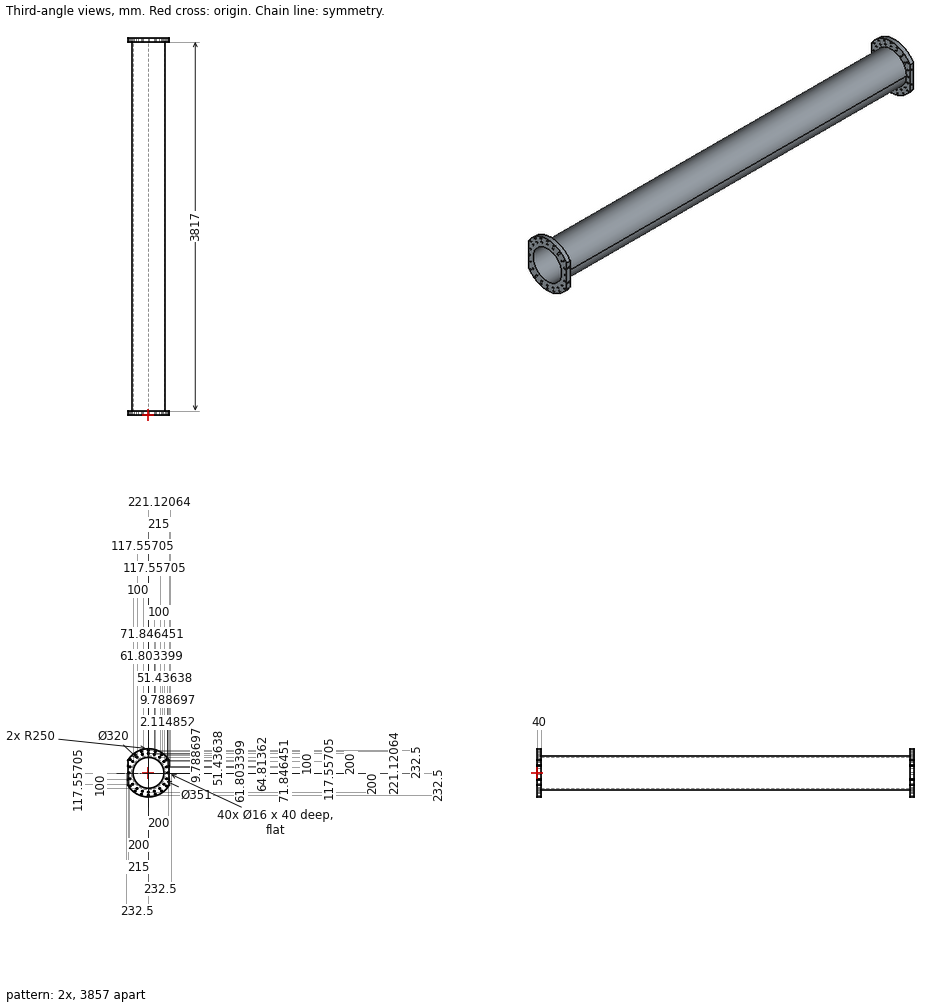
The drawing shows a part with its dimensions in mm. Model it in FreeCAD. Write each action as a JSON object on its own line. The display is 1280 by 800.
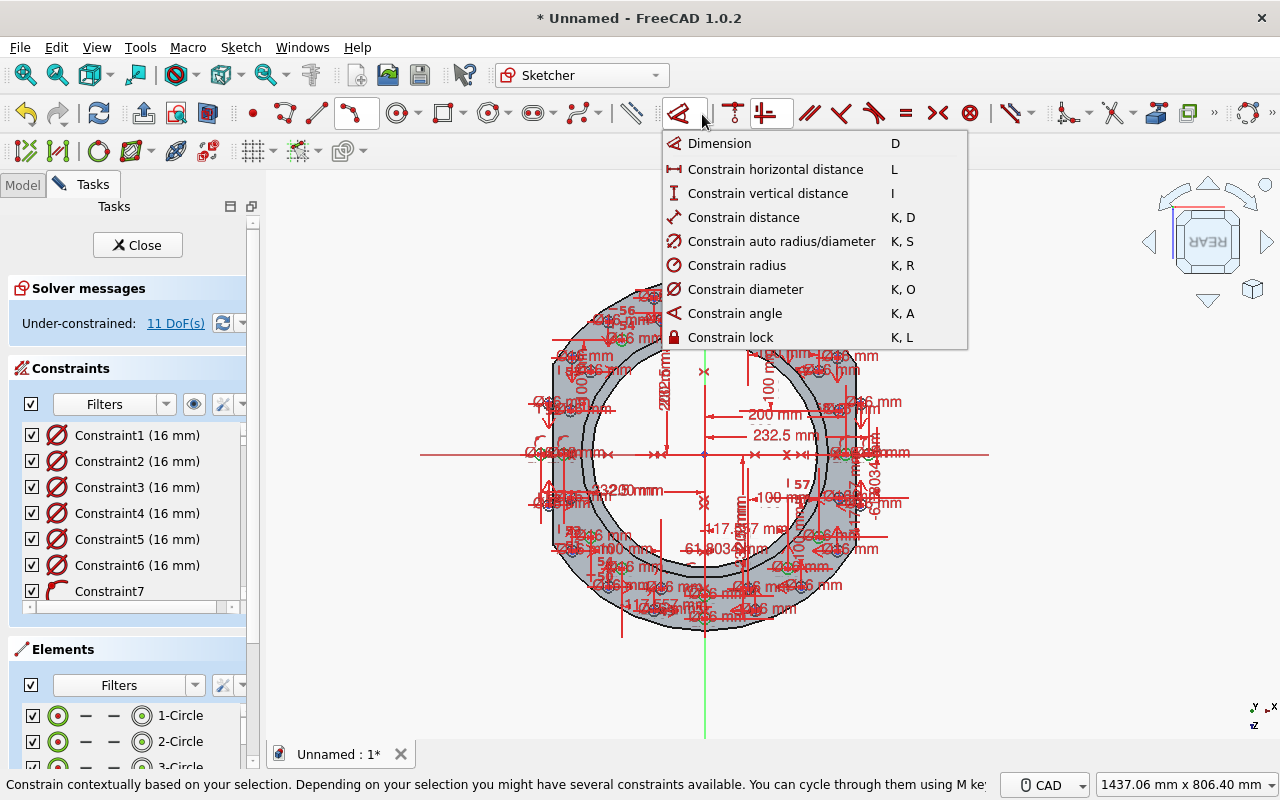
{"action": "left_click", "coordinate": [815, 193]}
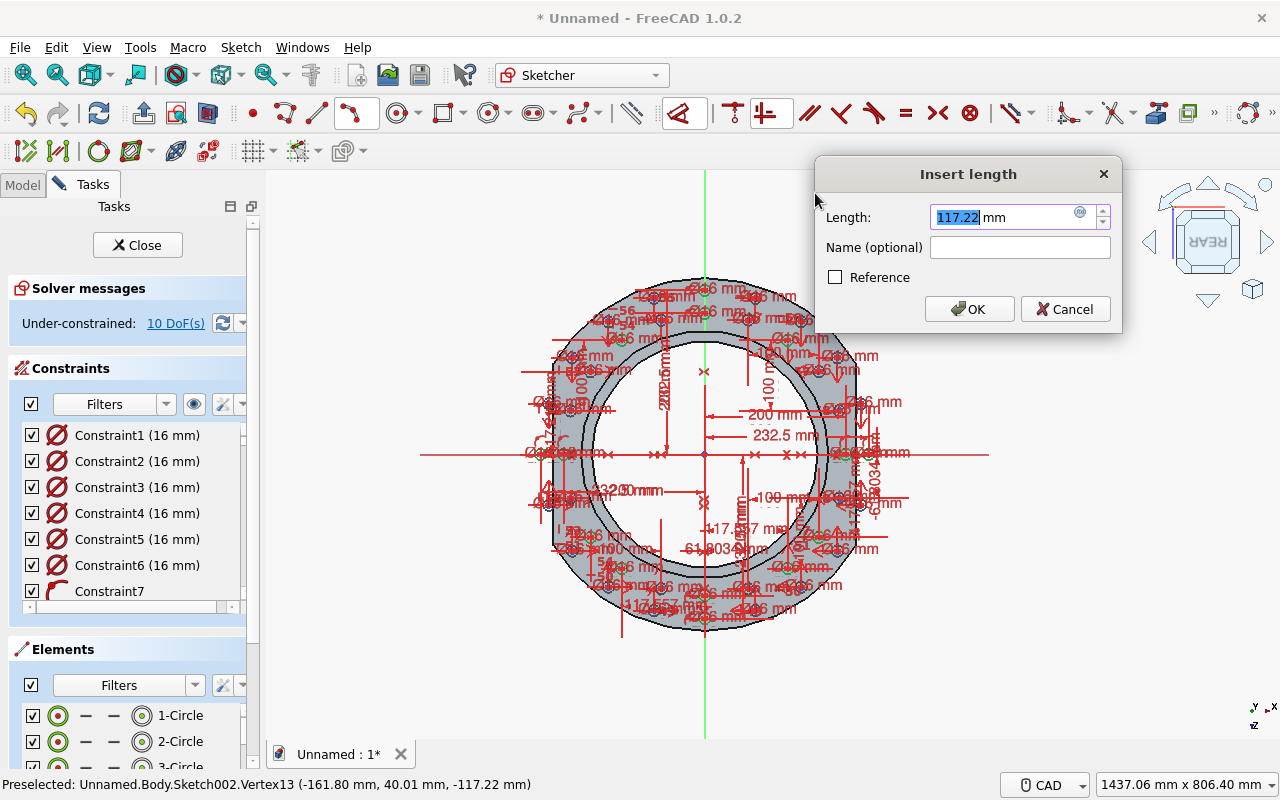
{"action": "type", "text": "117.55705"}
{"action": "key", "text": "Return"}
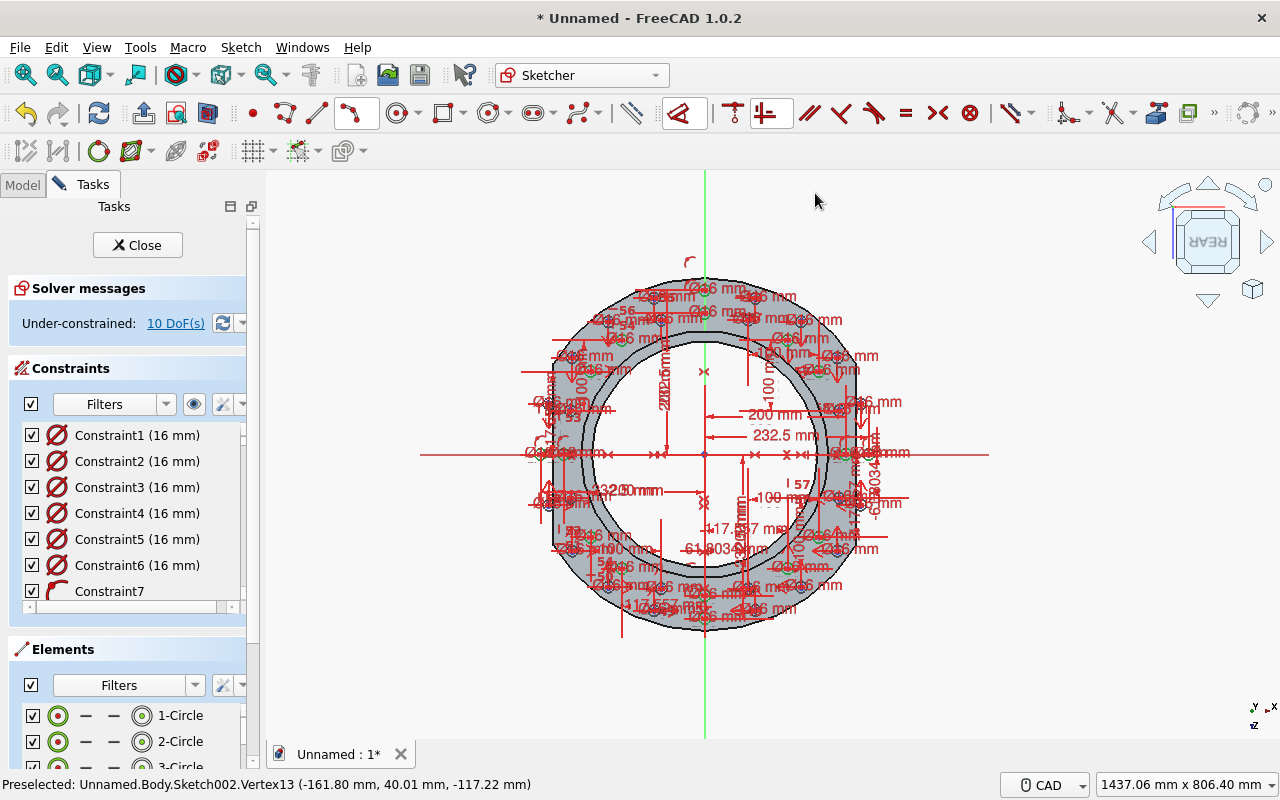
{"action": "left_click", "coordinate": [861, 505]}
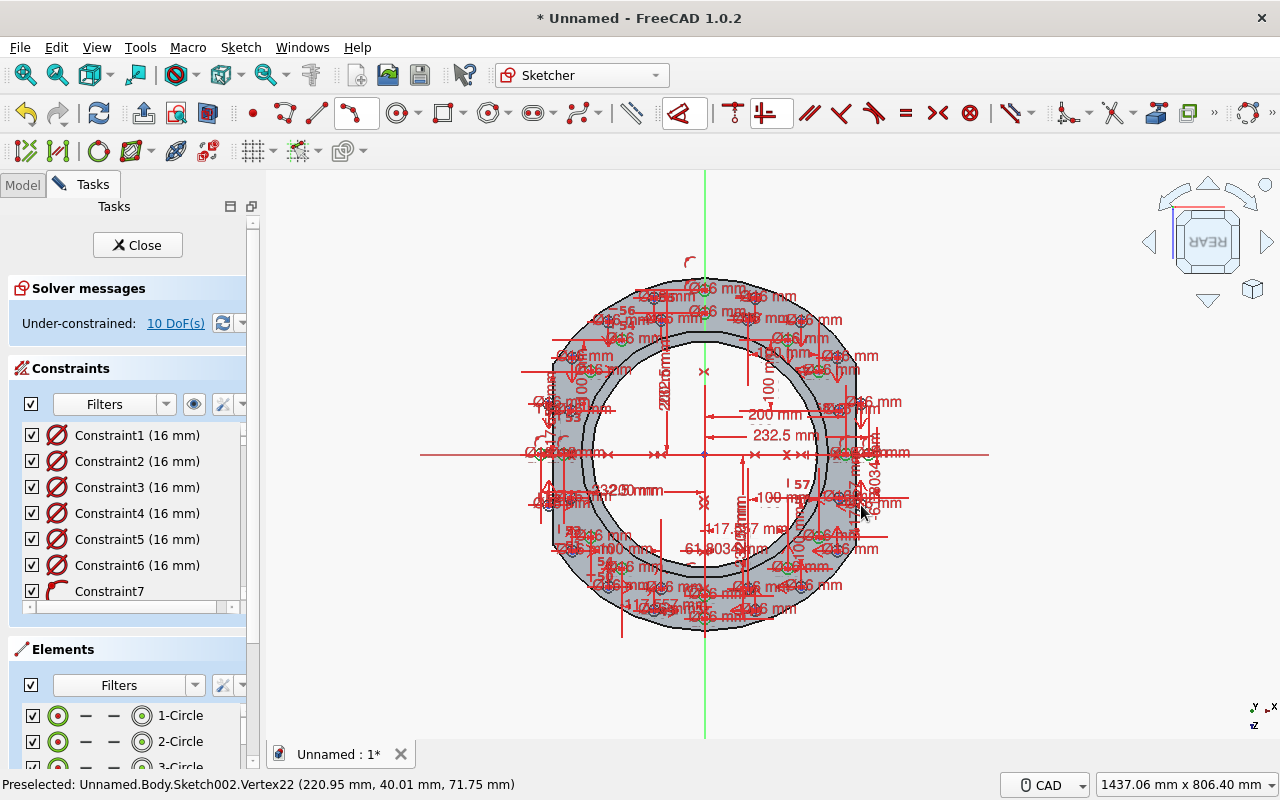
{"action": "left_click", "coordinate": [702, 114]}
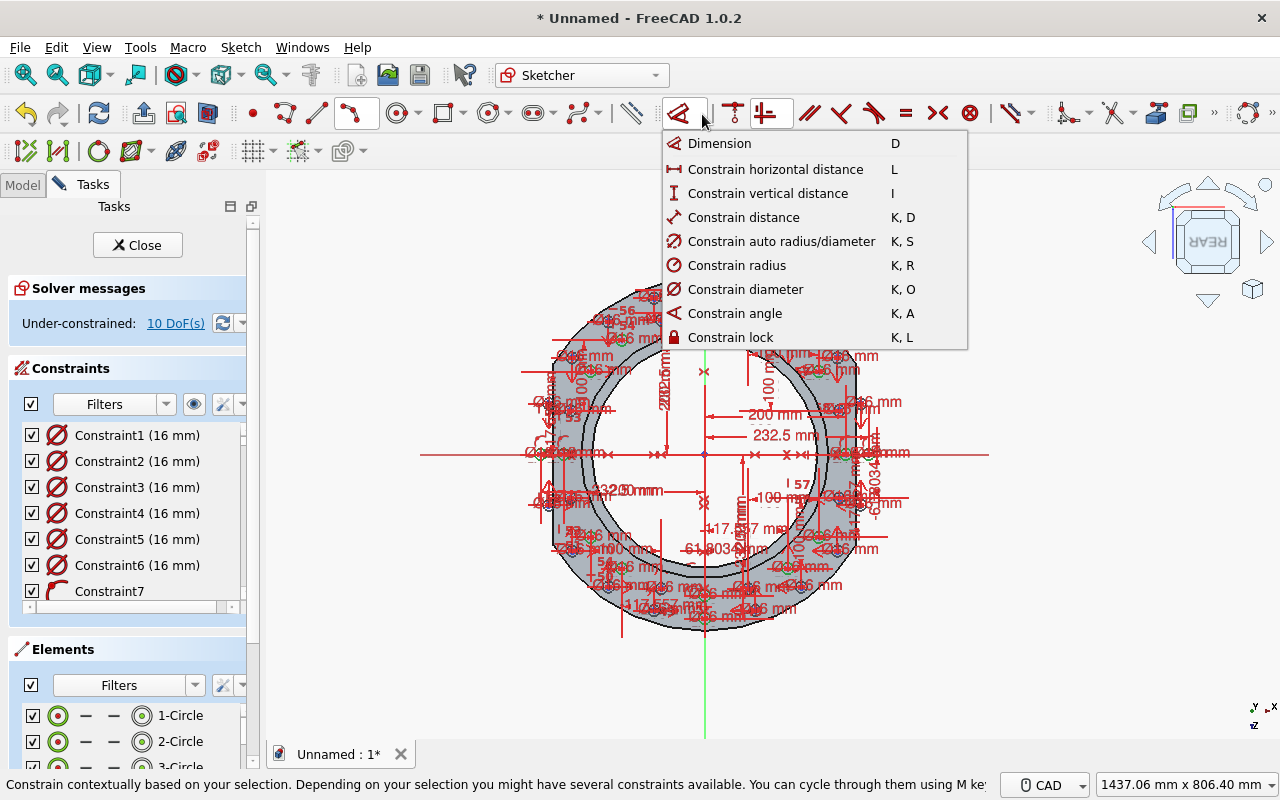
{"action": "left_click", "coordinate": [815, 169]}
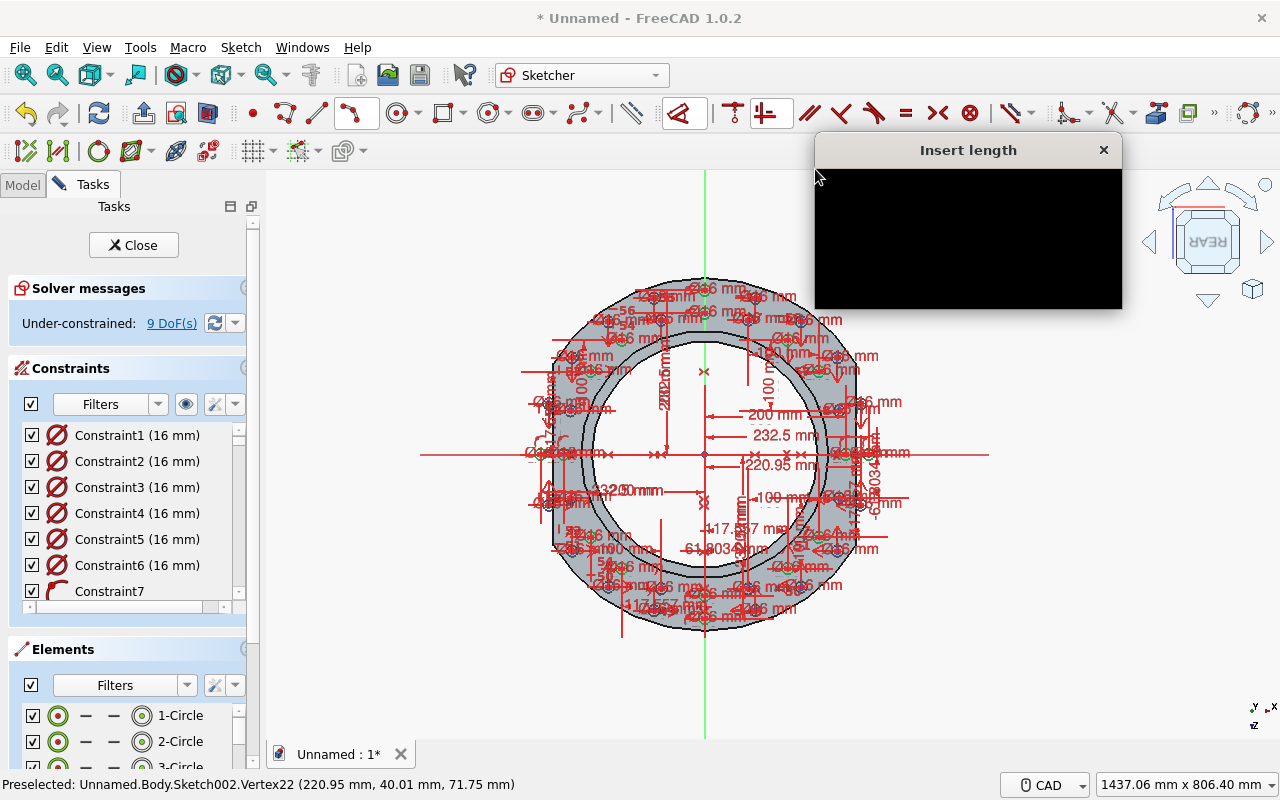
{"action": "type", "text": "221.12064"}
{"action": "key", "text": "Return"}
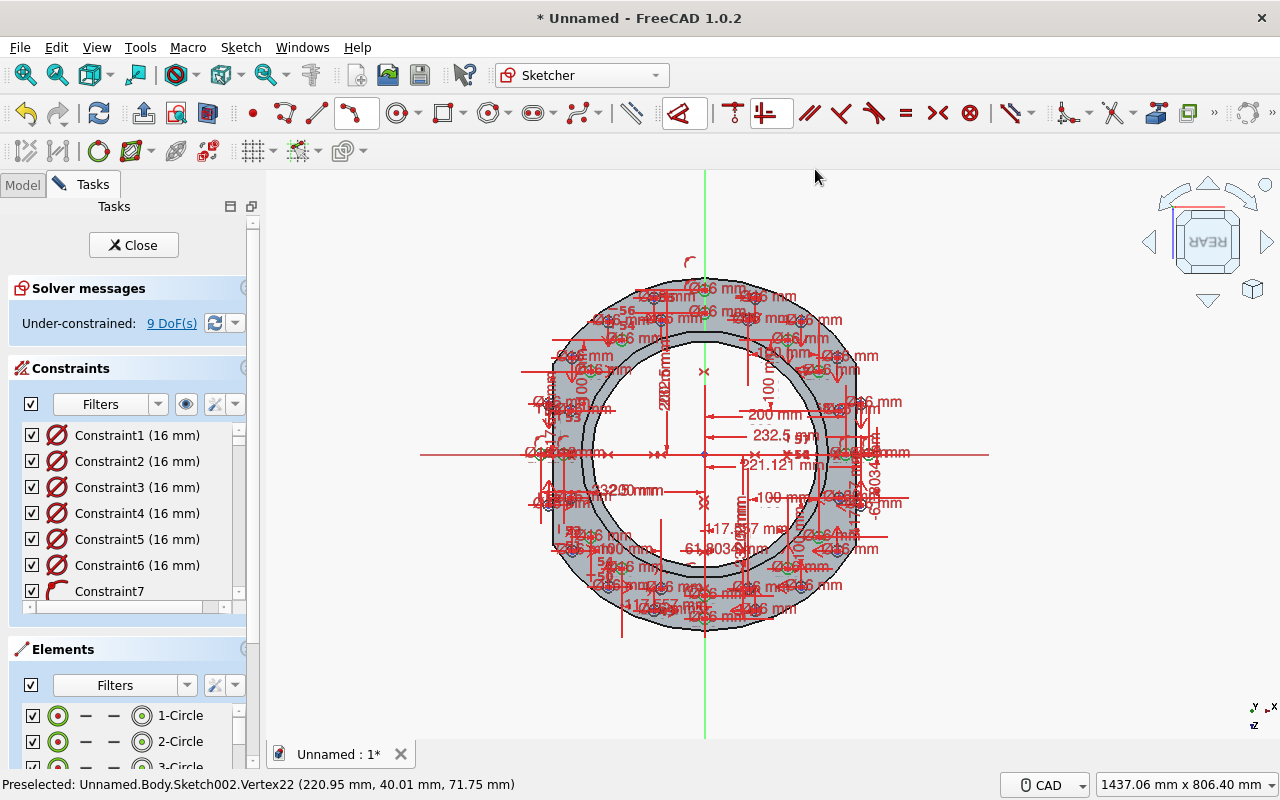
{"action": "left_click", "coordinate": [861, 505]}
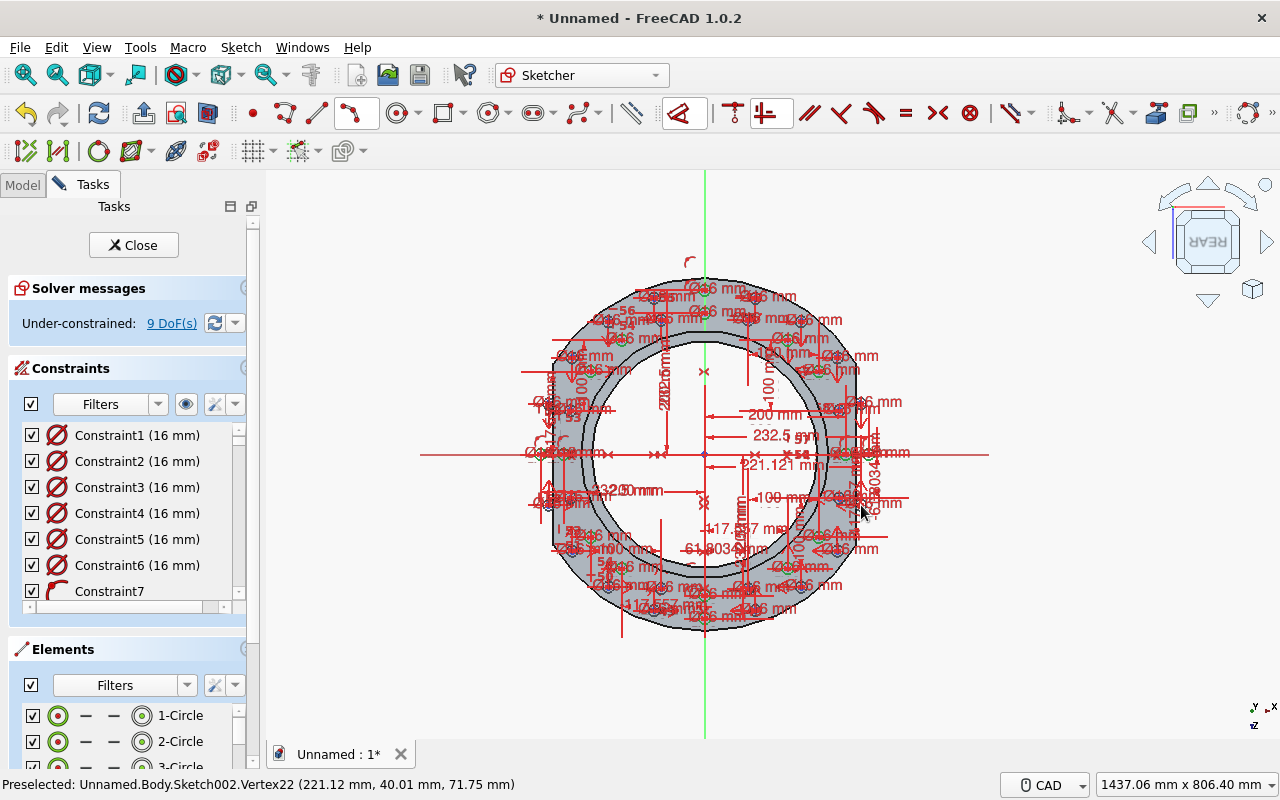
{"action": "left_click", "coordinate": [702, 114]}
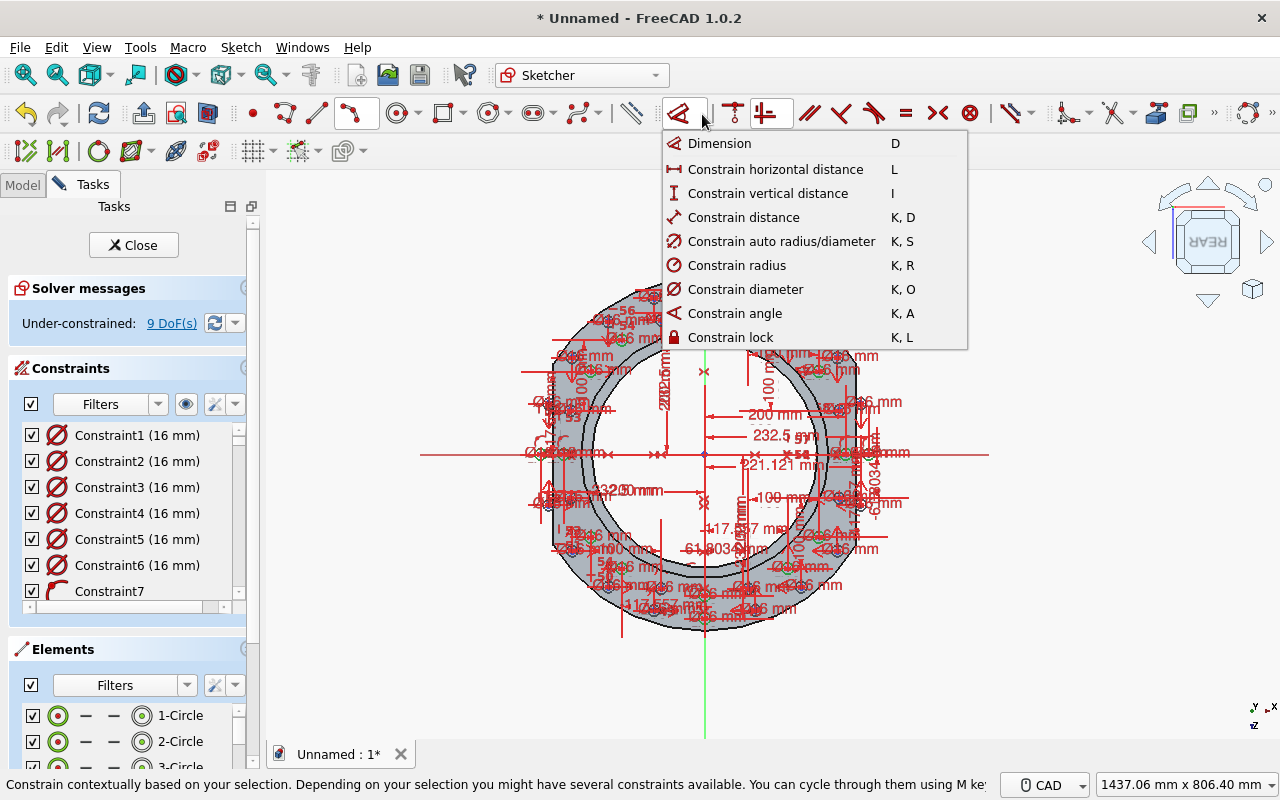
{"action": "left_click", "coordinate": [815, 193]}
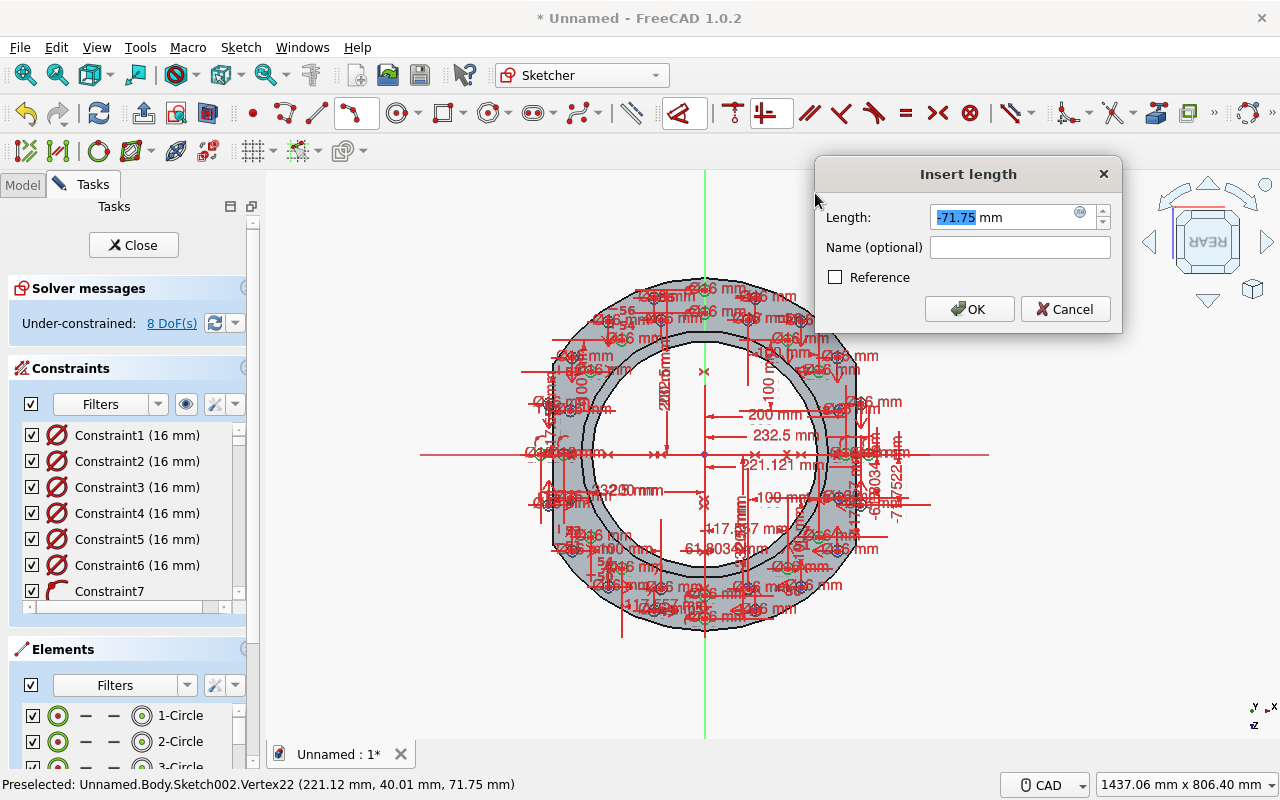
{"action": "type", "text": "-71.846451"}
{"action": "key", "text": "Return"}